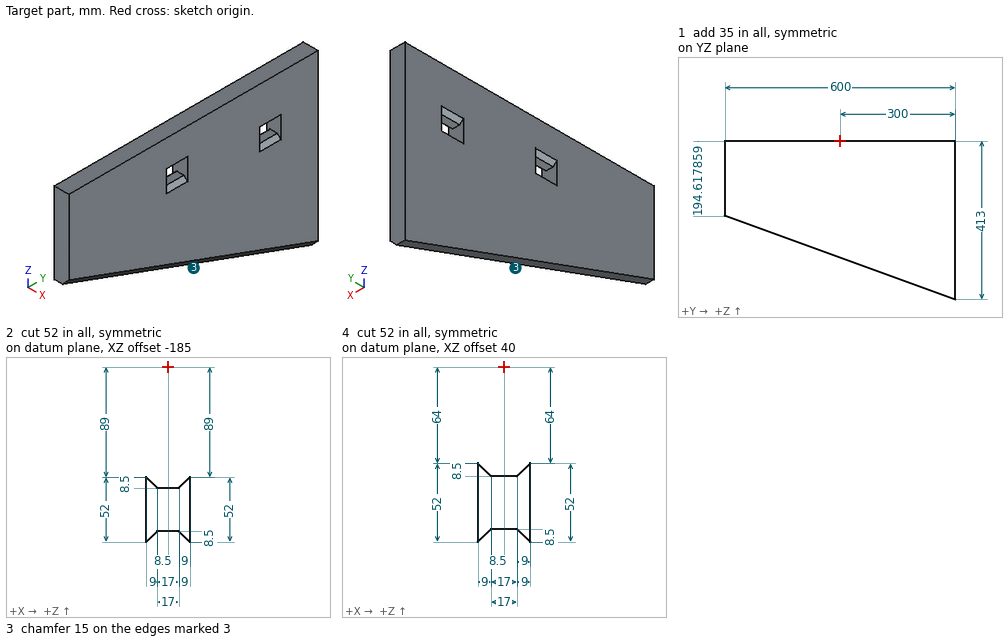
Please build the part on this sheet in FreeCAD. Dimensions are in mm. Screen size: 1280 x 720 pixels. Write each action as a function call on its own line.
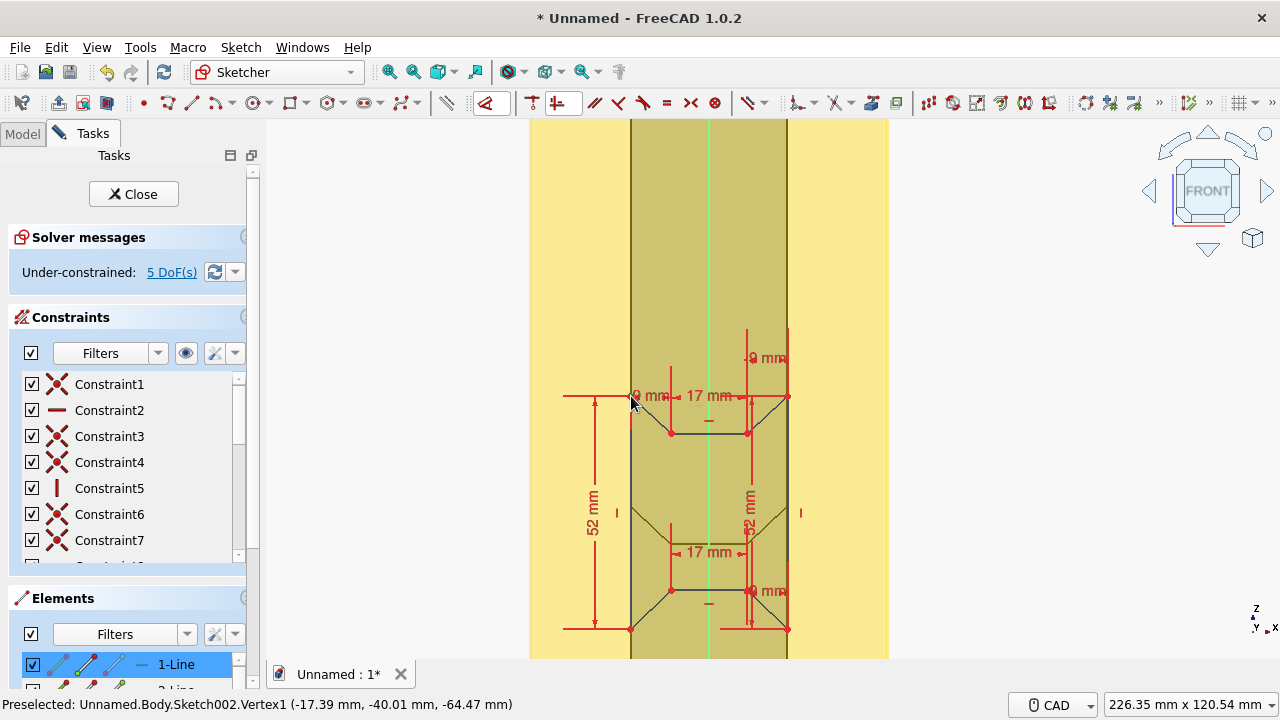
key(i)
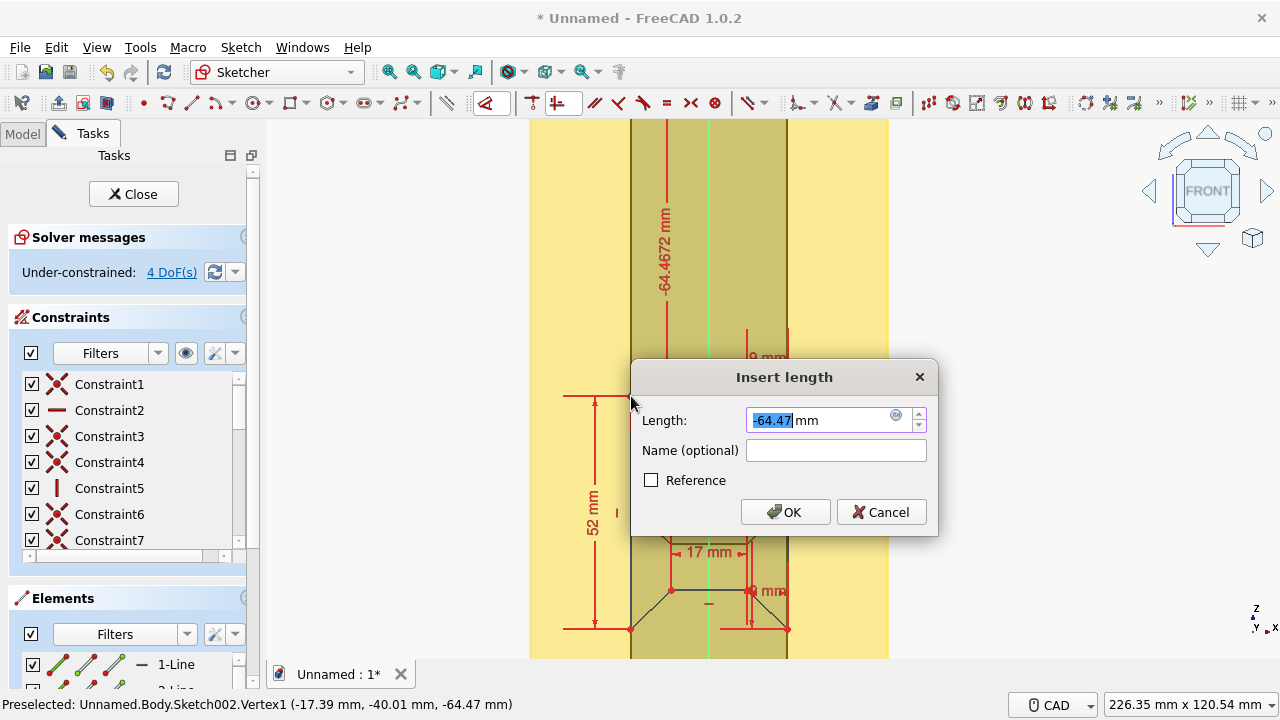
text(-64)
key(Return)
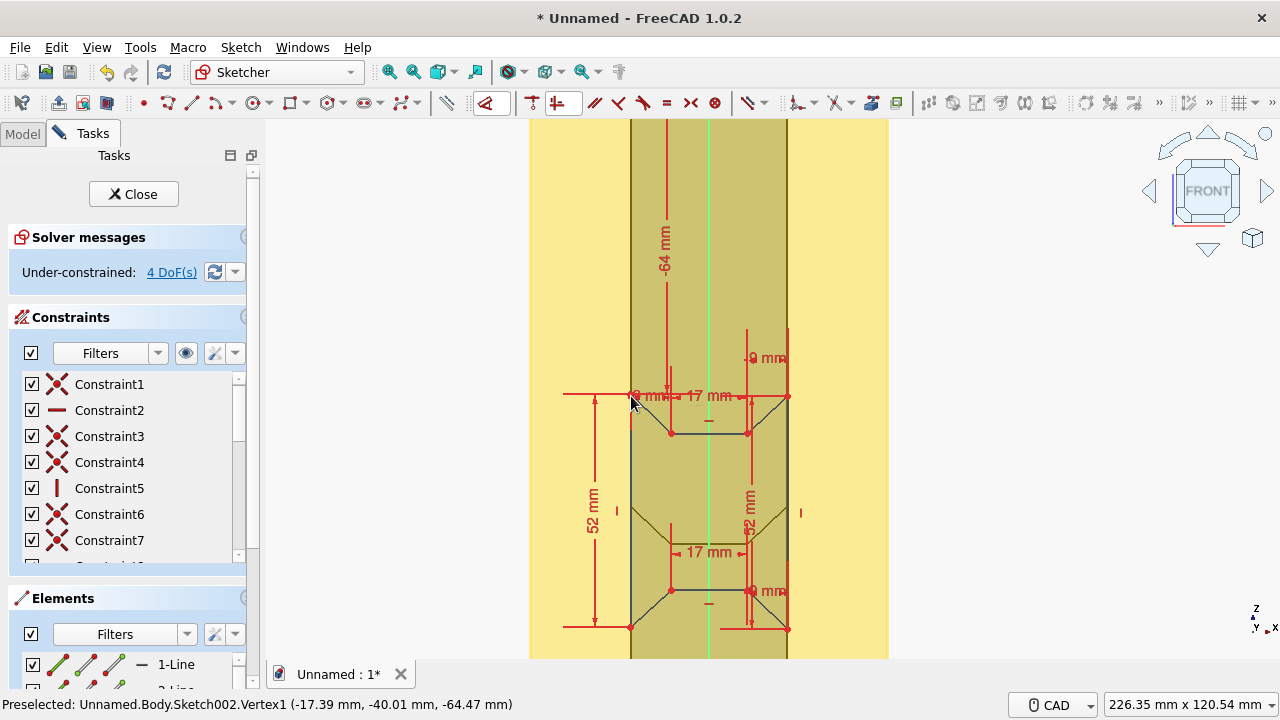
click(788, 396)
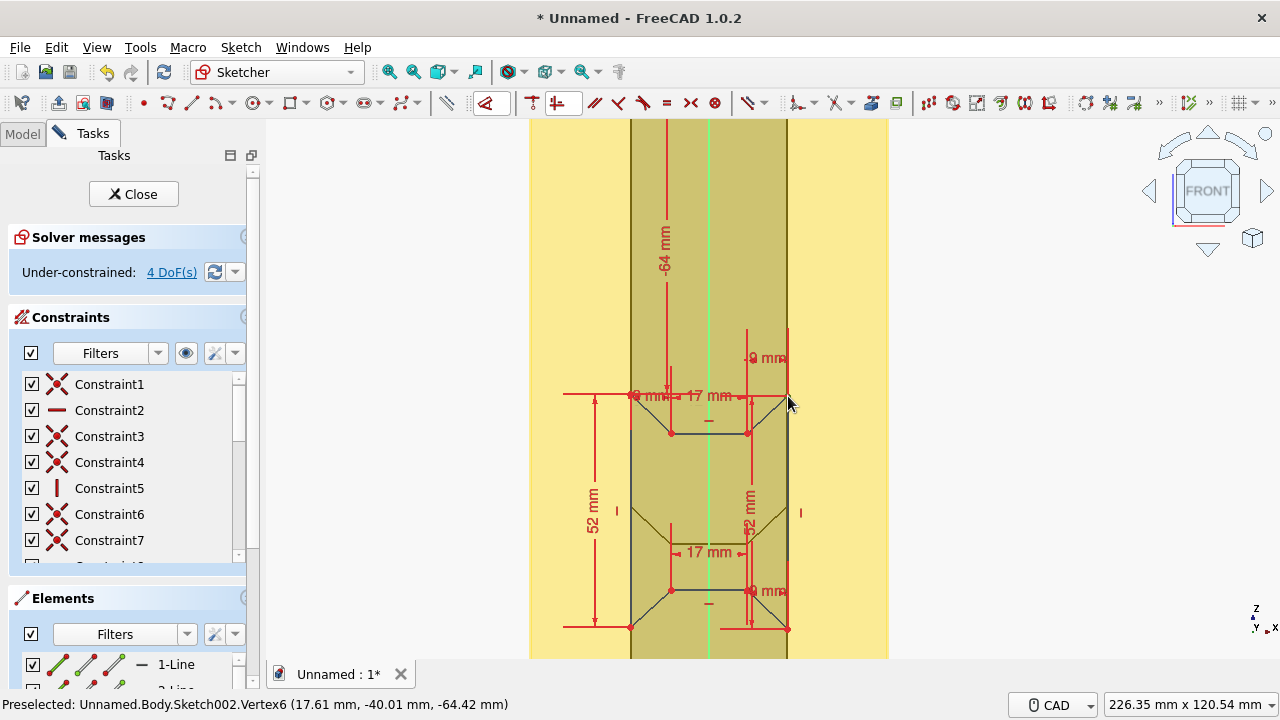
key(i)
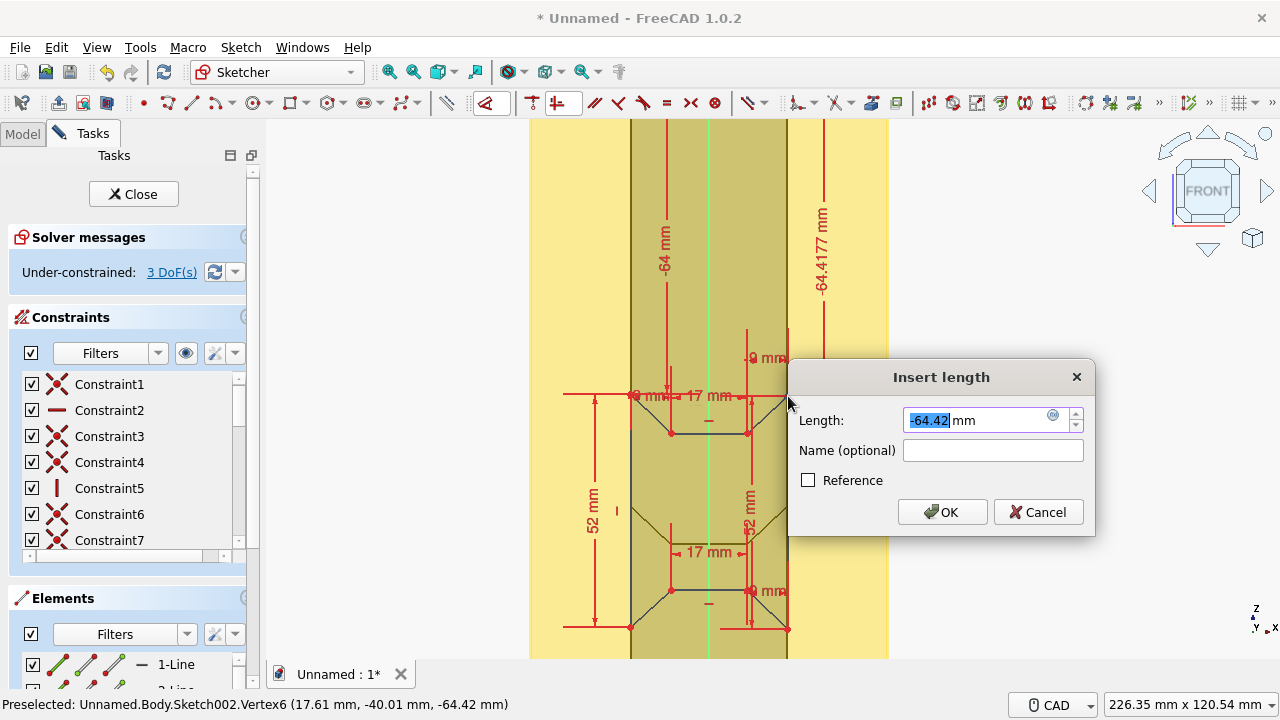
text(-64)
key(Return)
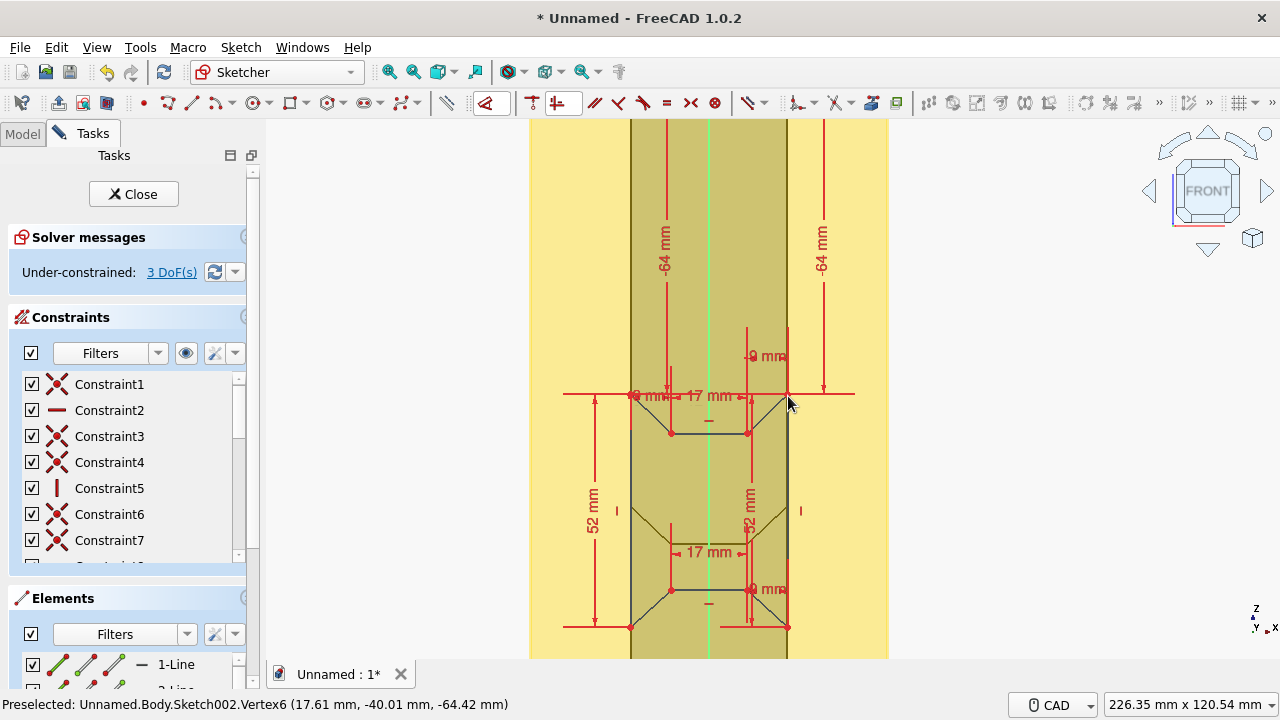
click(671, 434)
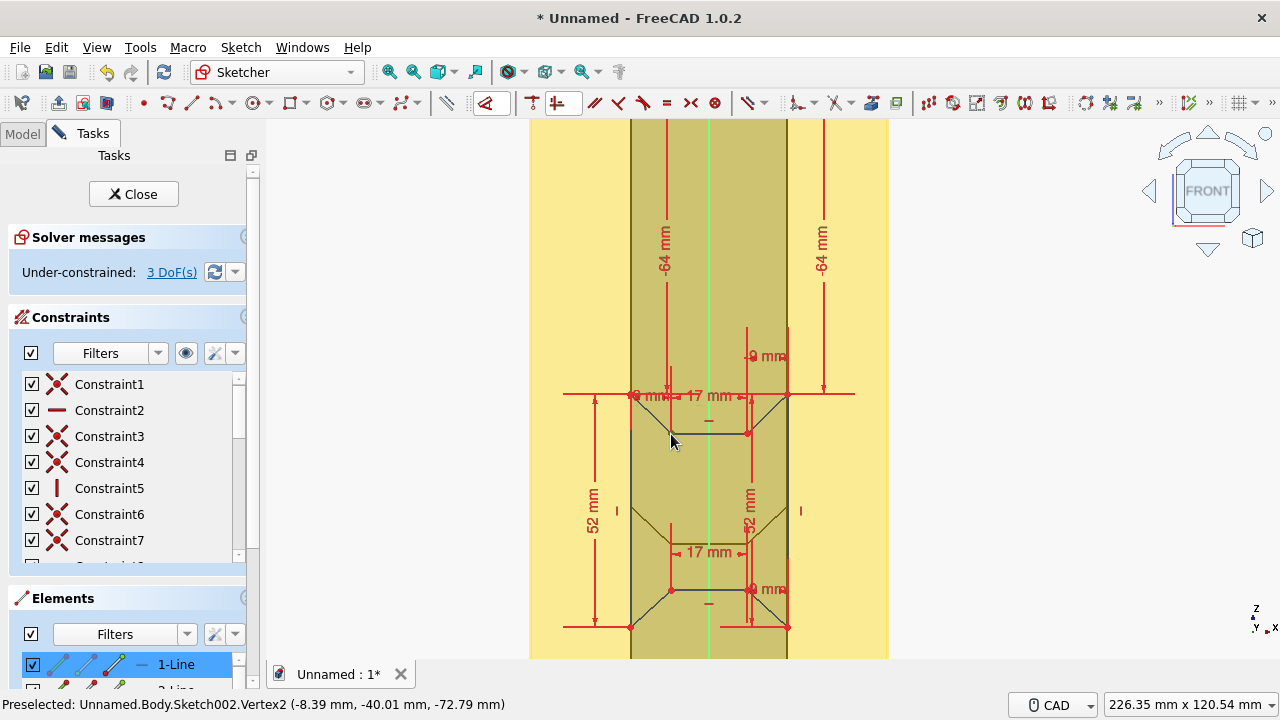
key(l)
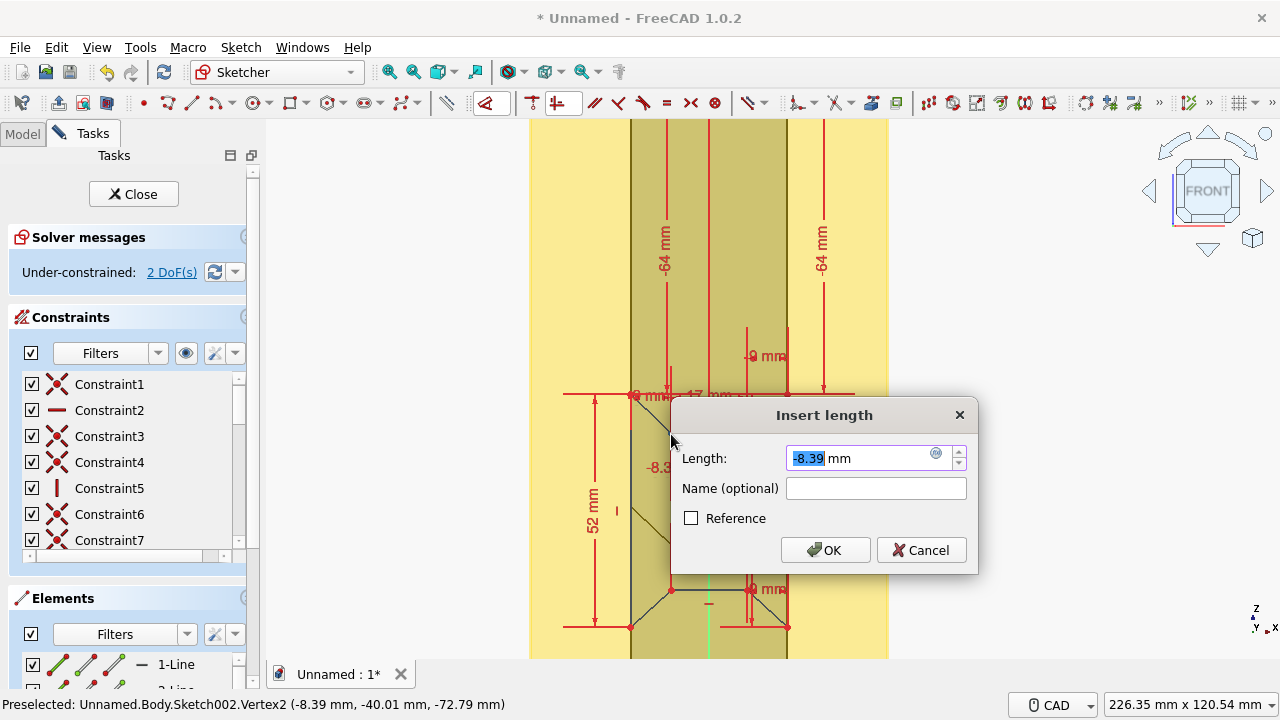
text(-8.5)
key(Return)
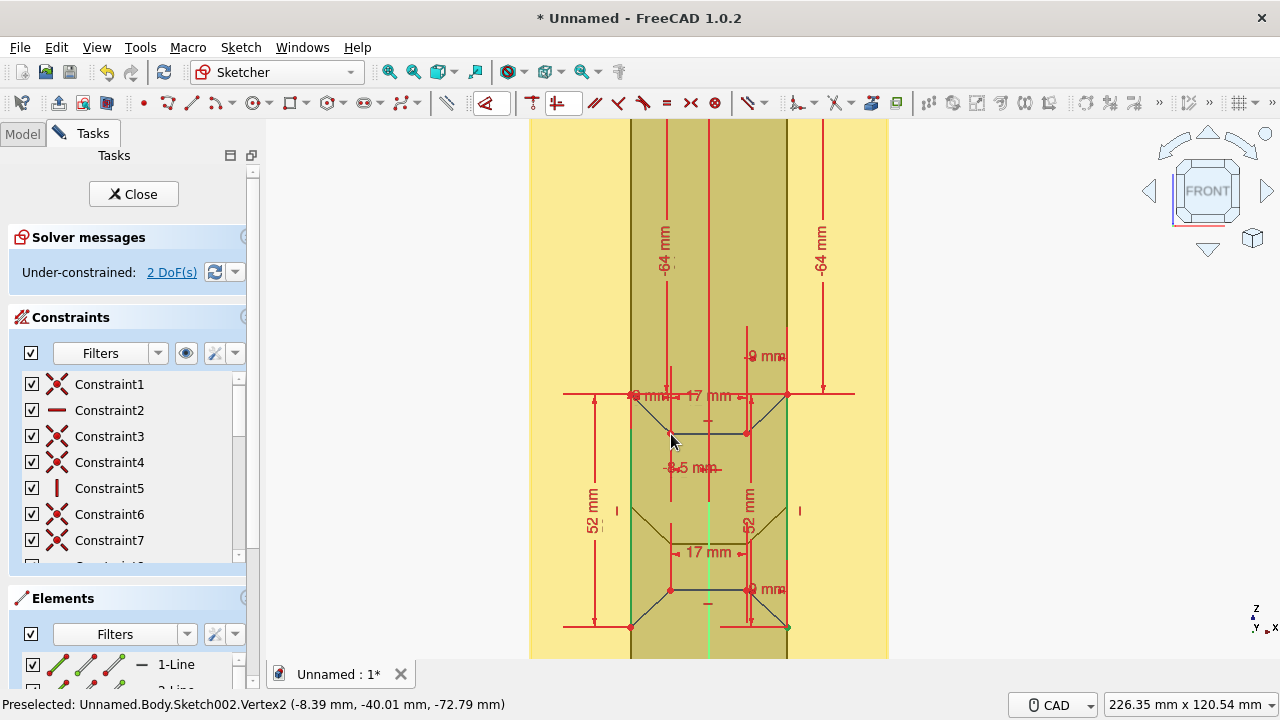
click(643, 406)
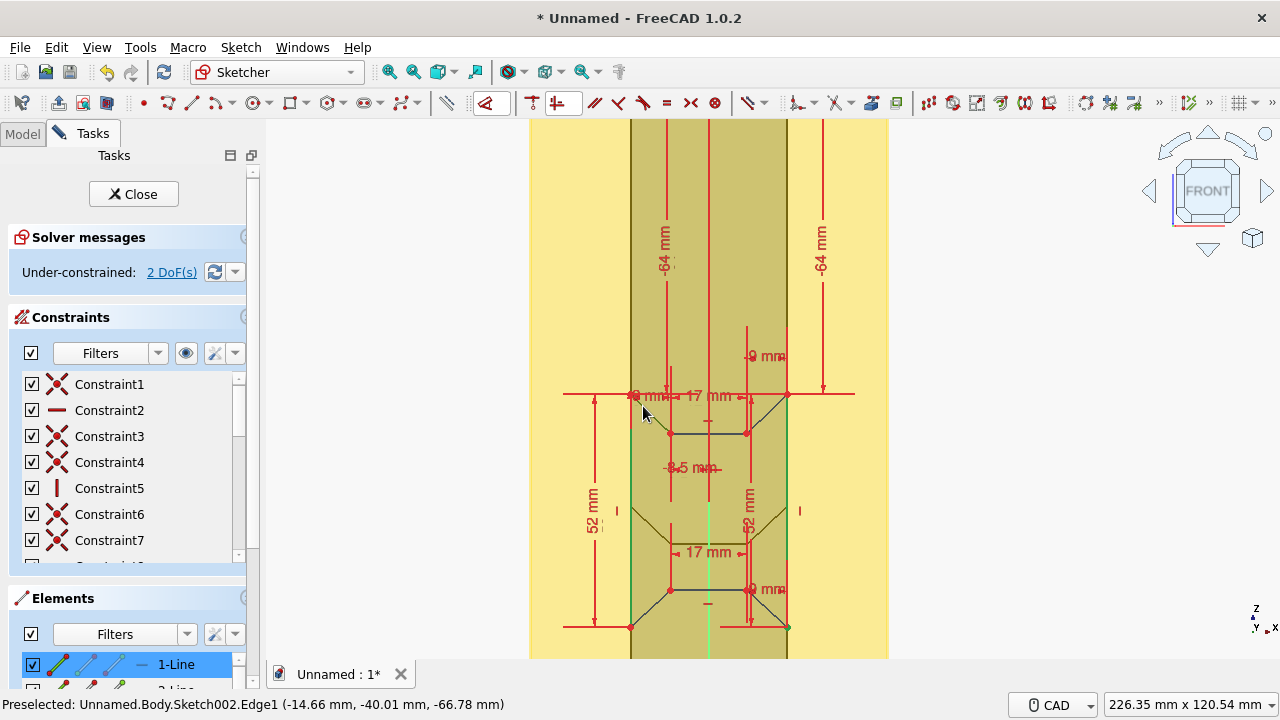
key(i)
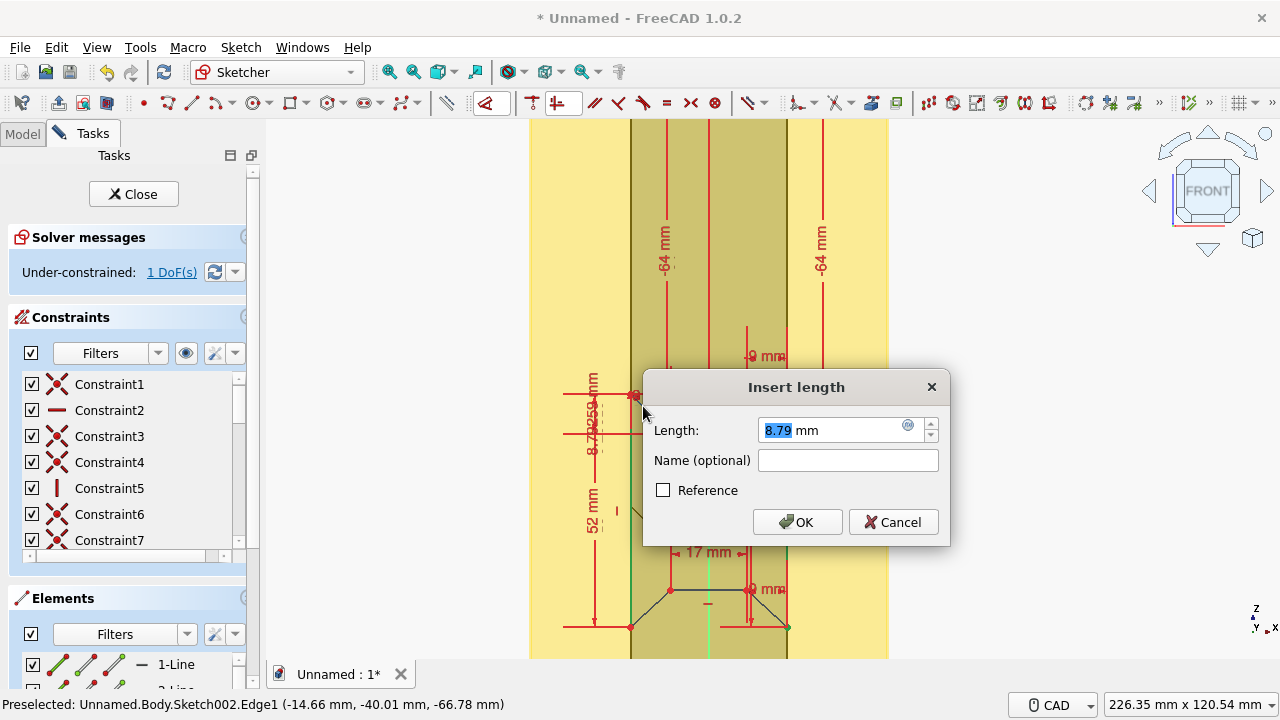
text(8.5)
key(Return)